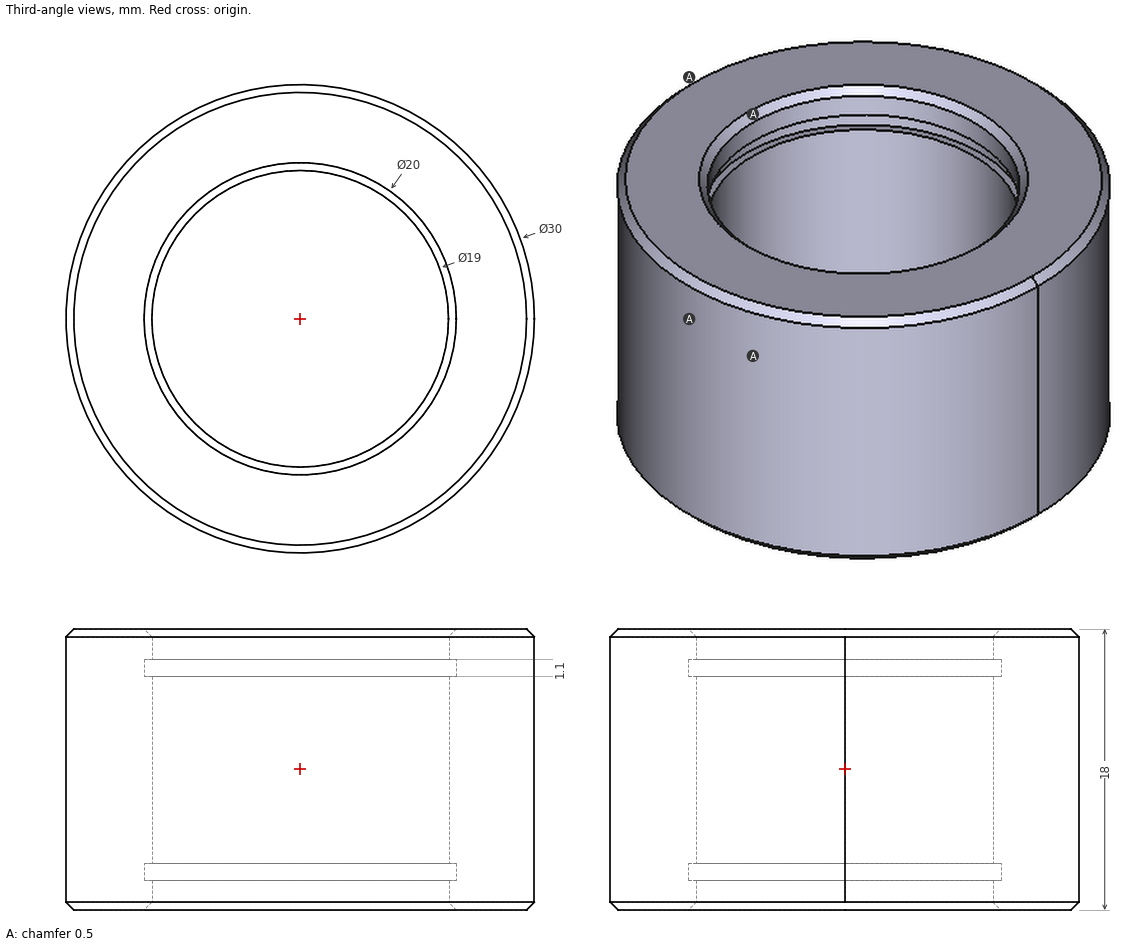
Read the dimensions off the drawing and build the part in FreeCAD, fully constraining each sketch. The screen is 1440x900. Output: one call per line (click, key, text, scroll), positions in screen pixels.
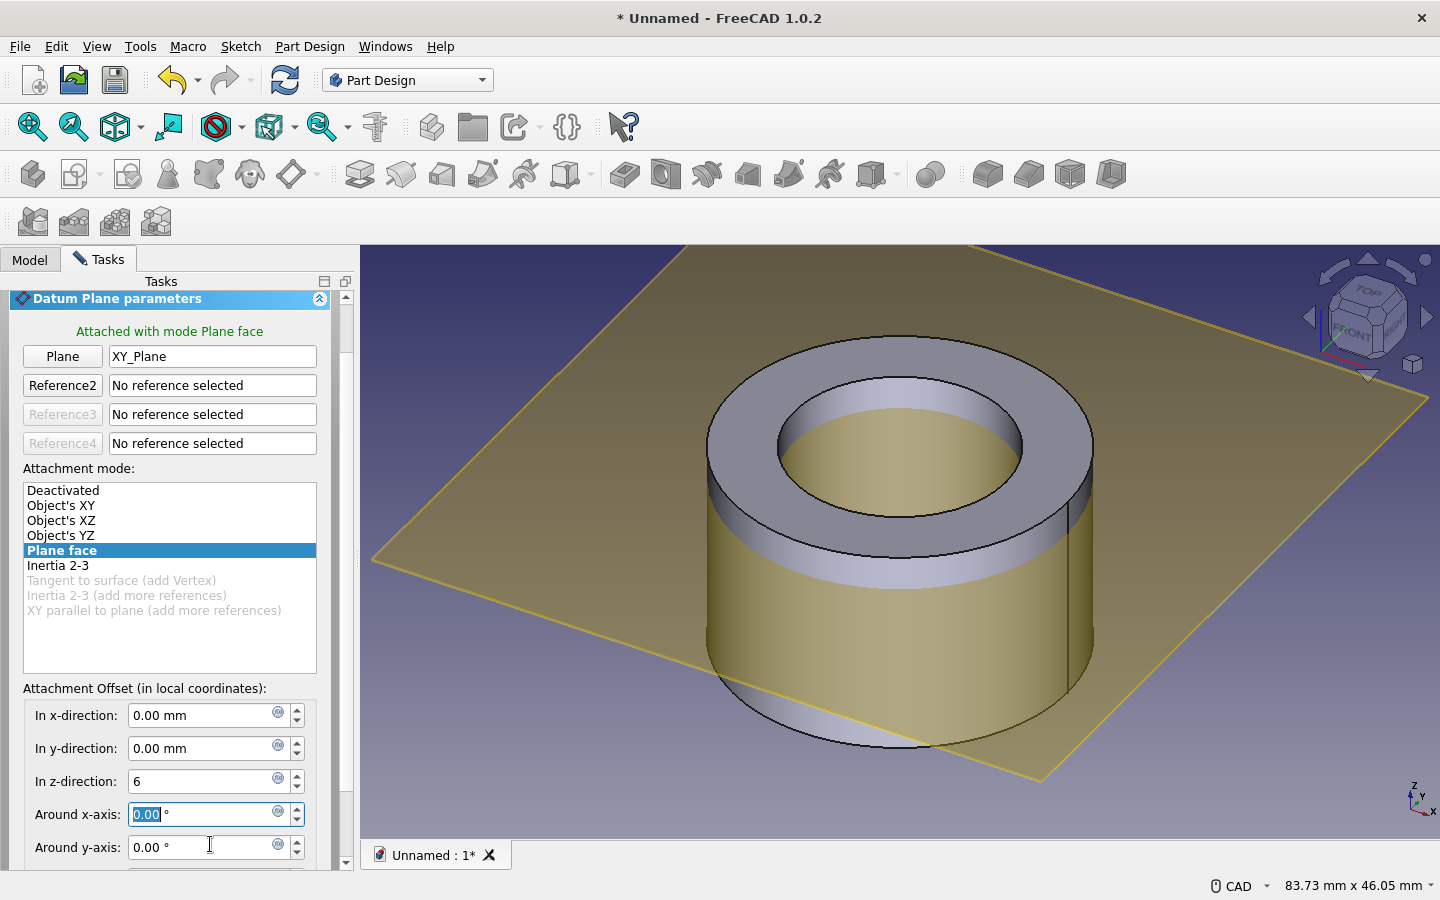
scroll(346, 580, up, 2)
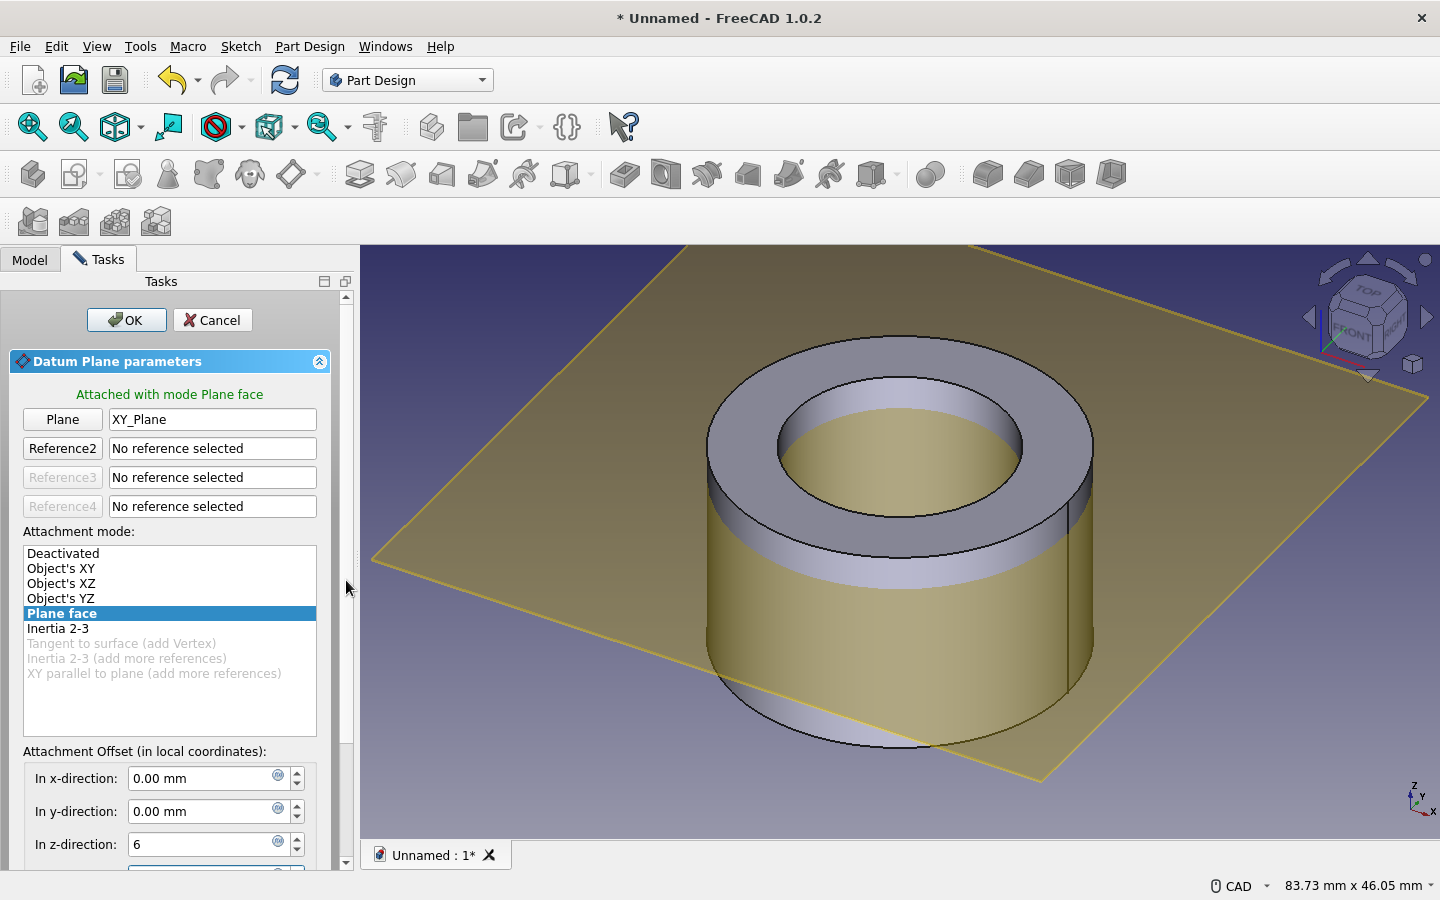
click(127, 320)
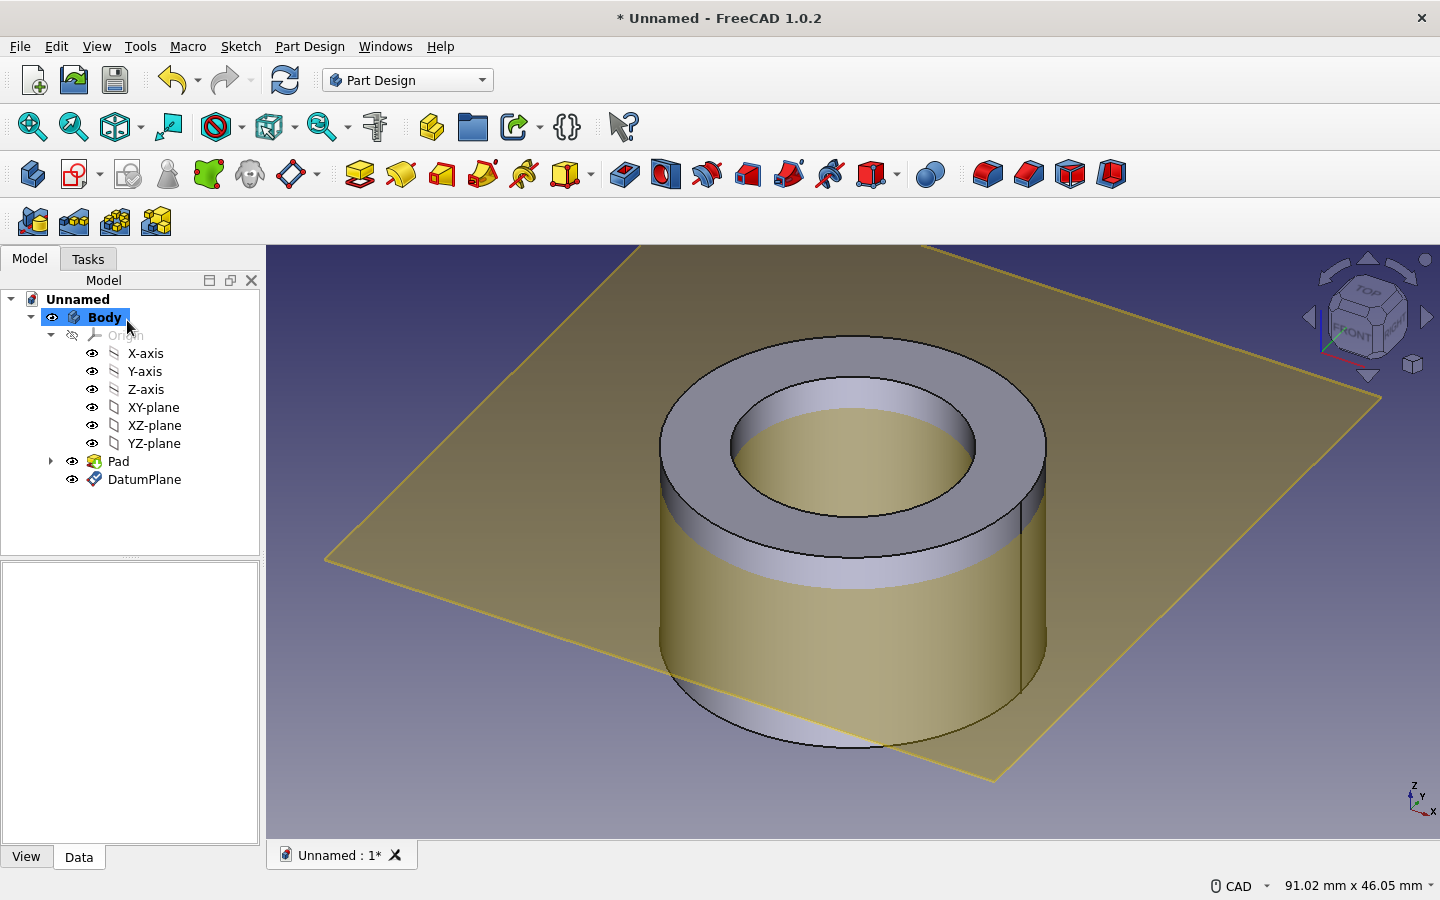
click(117, 479)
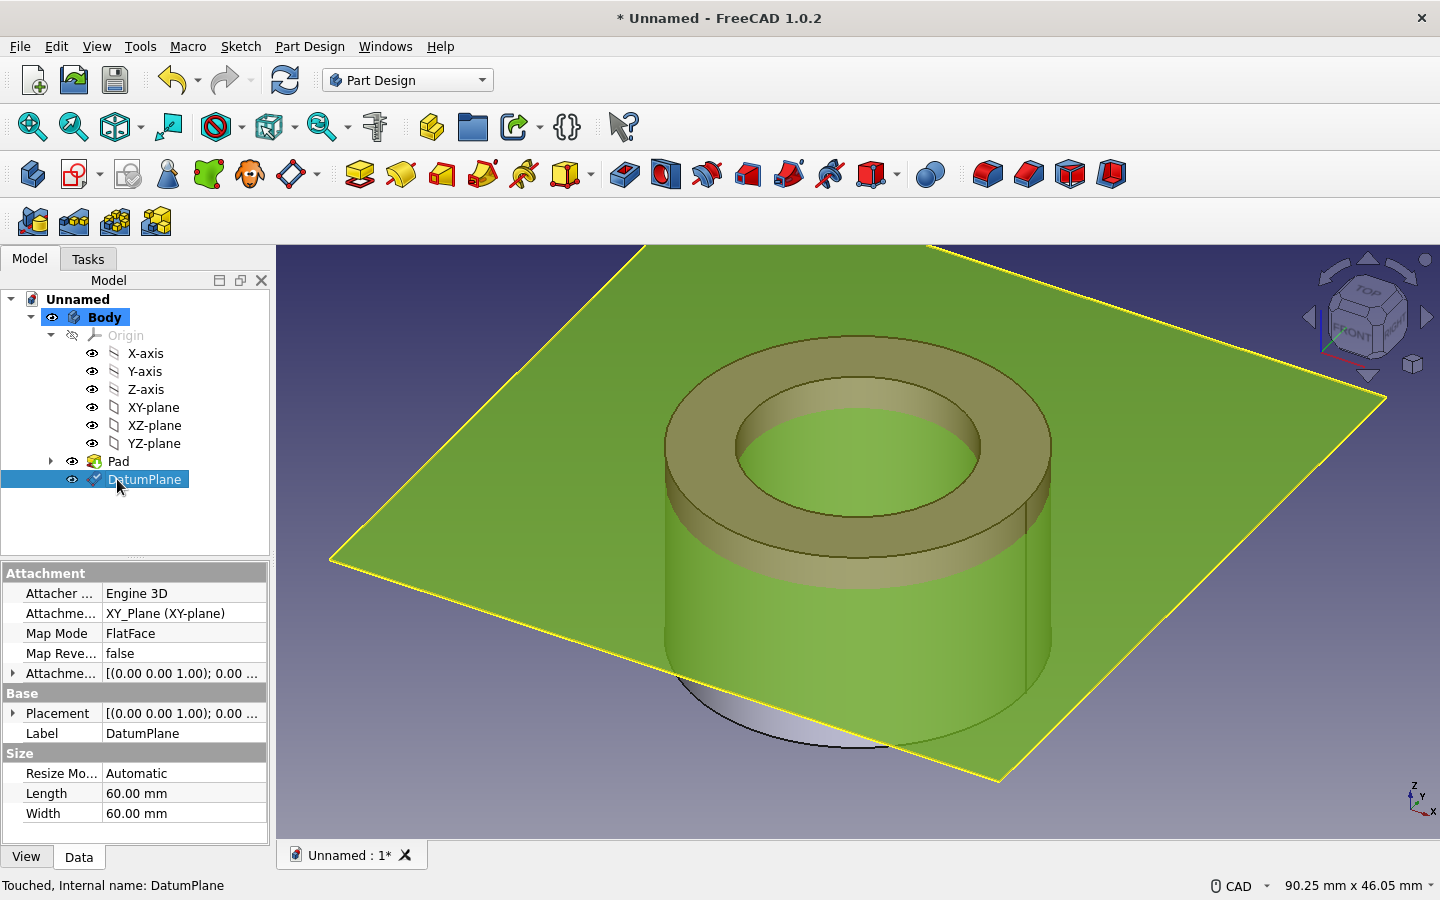
click(74, 174)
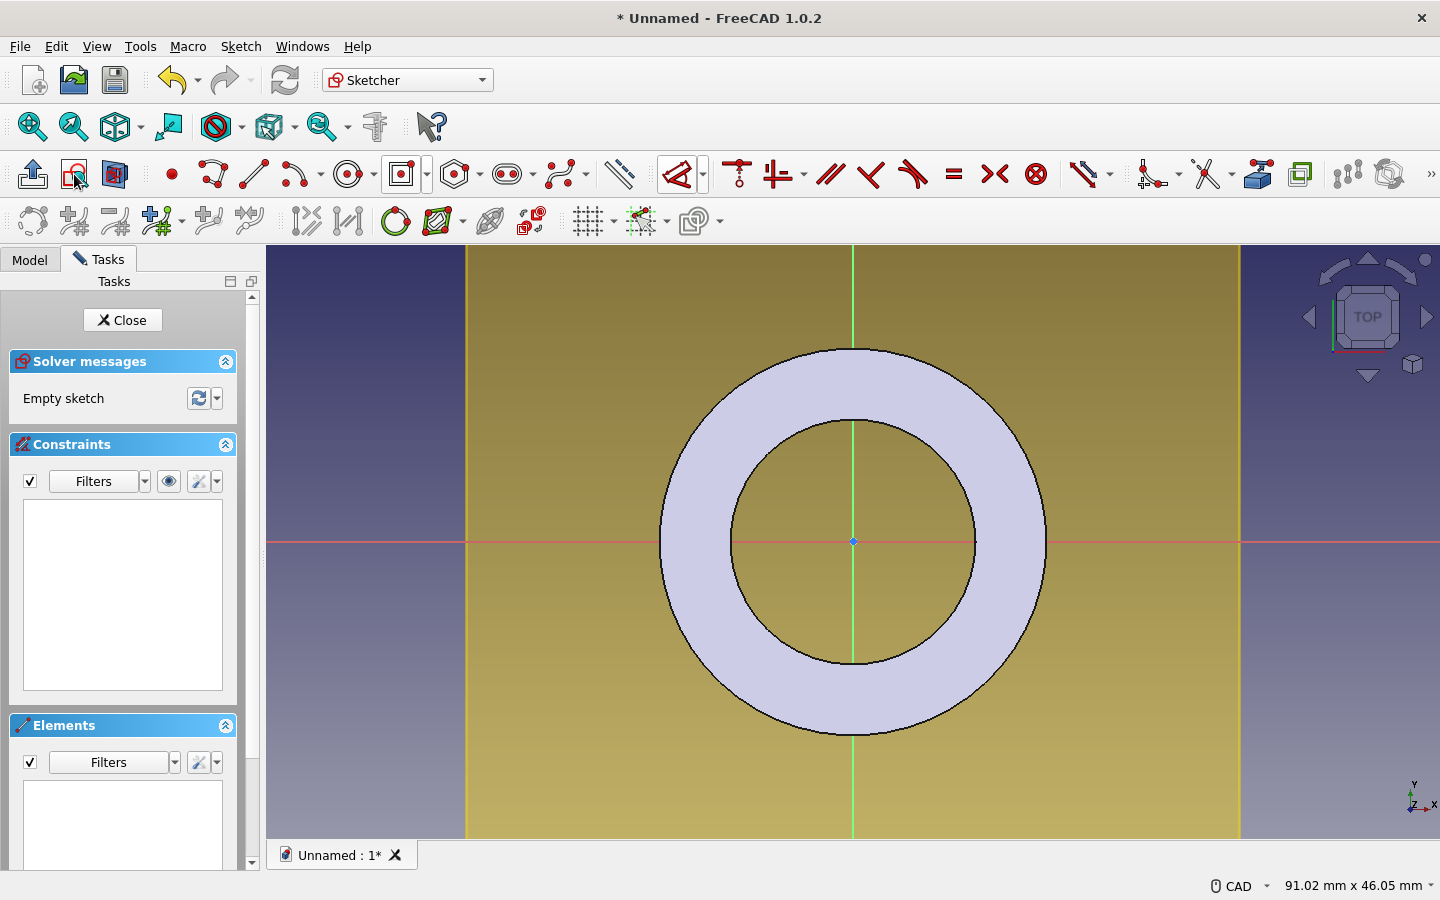
key(q)
key(s)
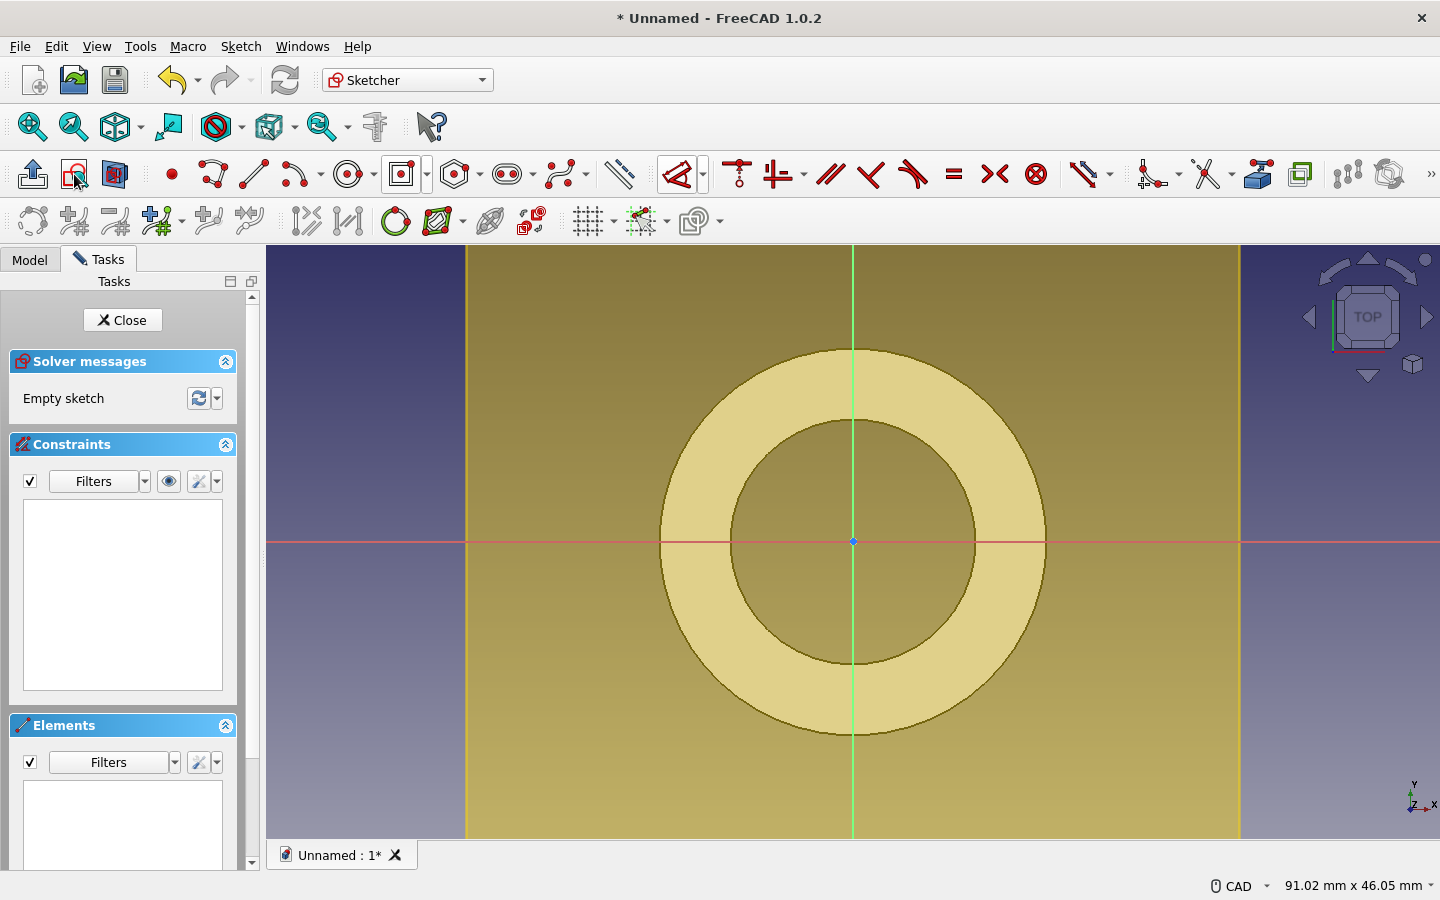
scroll(992, 542, up, 2)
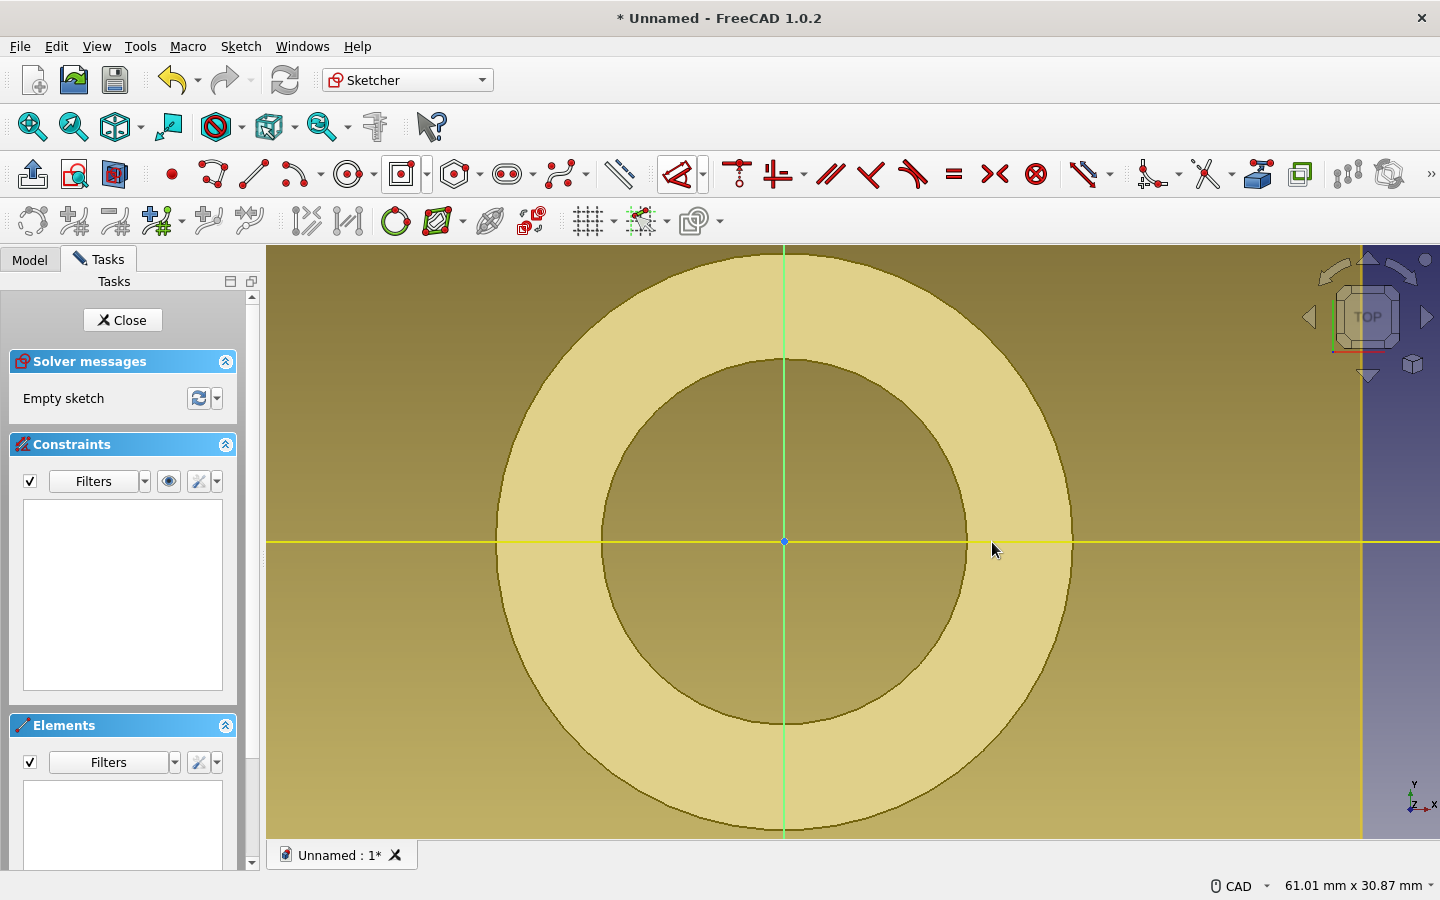
click(348, 174)